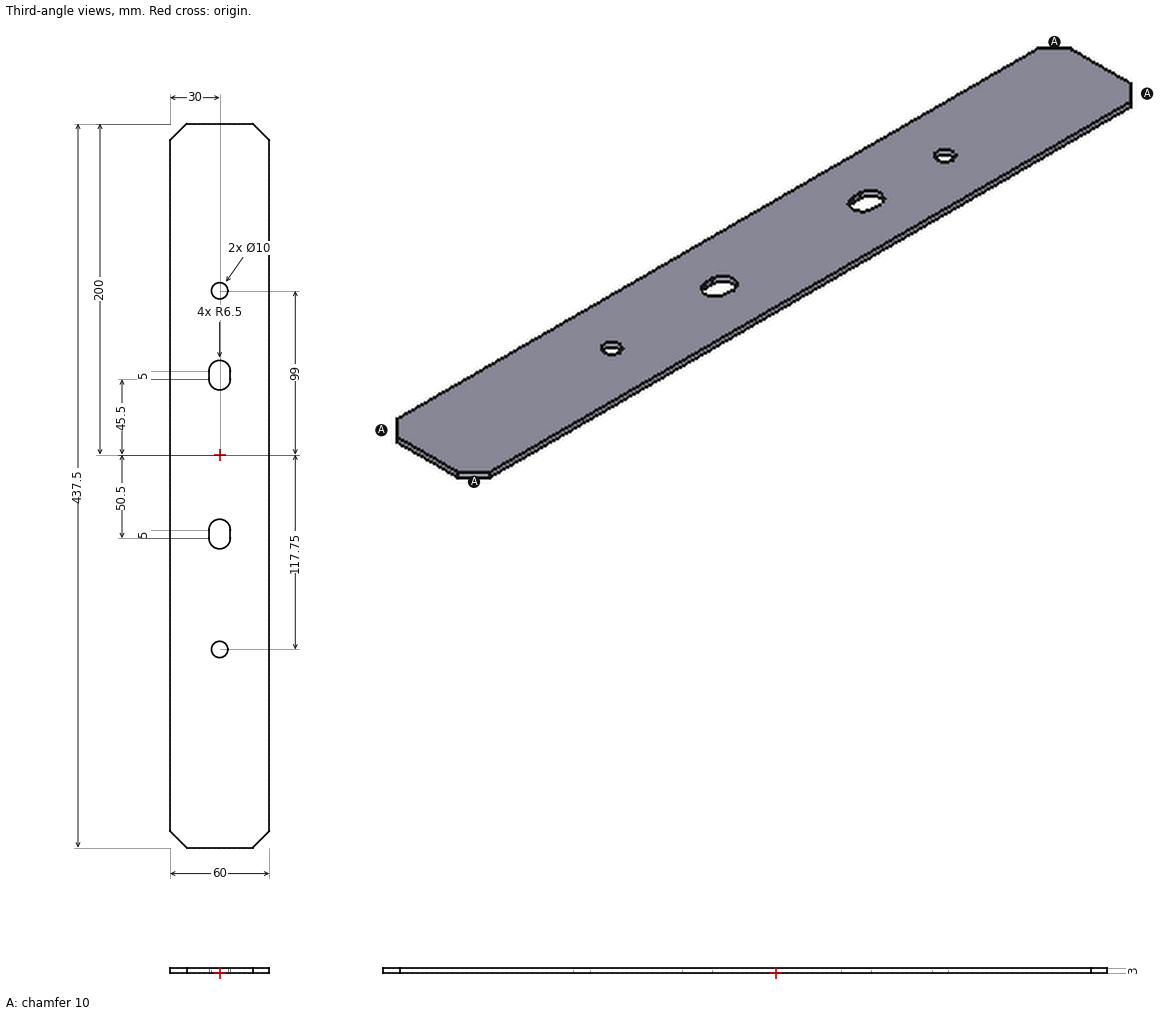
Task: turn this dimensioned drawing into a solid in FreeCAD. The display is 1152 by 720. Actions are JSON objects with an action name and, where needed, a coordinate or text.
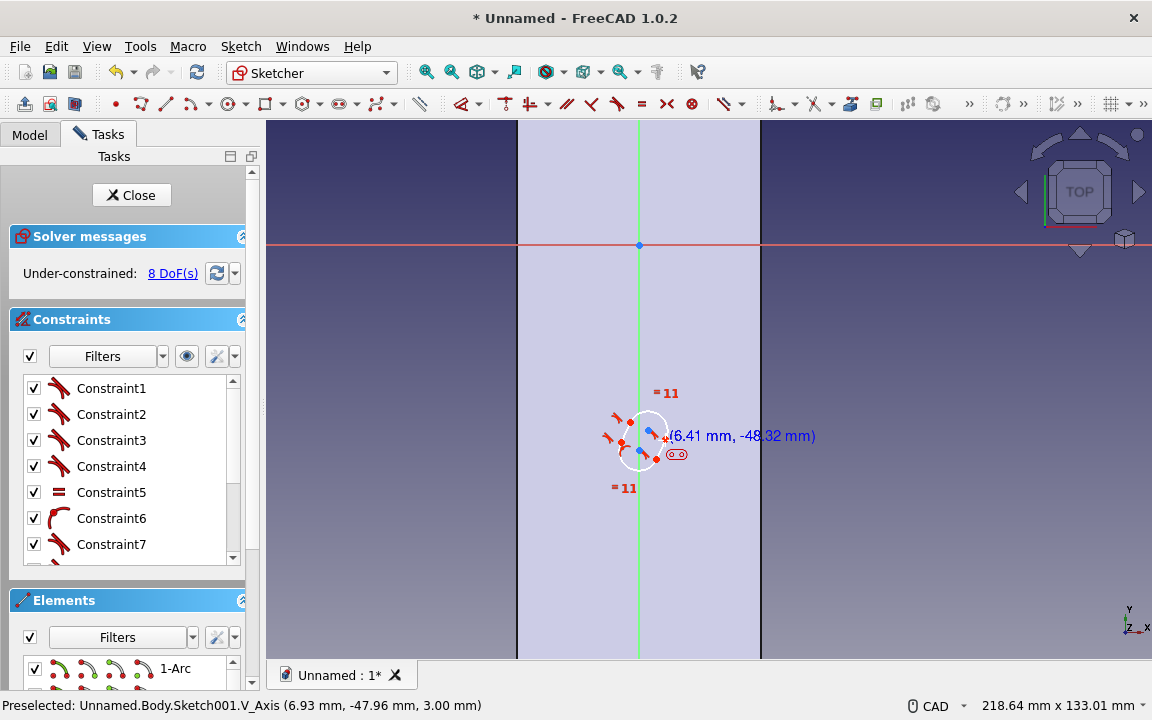
{"action": "key", "text": "g c"}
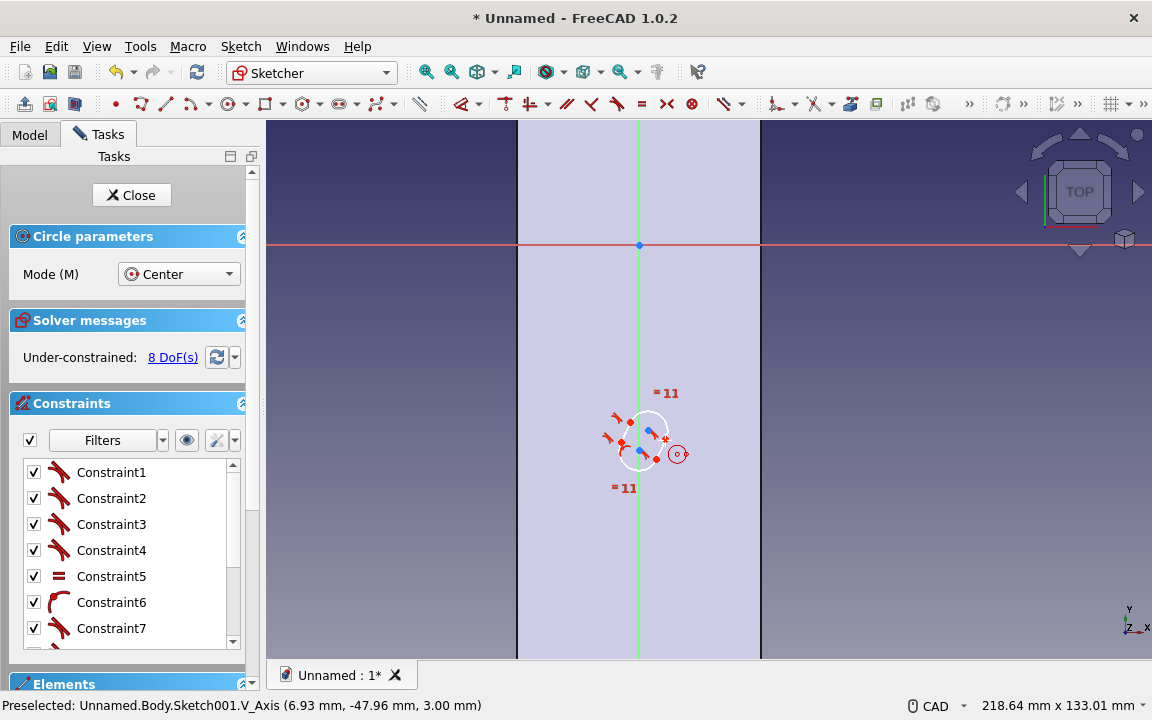
{"action": "scroll", "coordinate": [641, 451], "scroll_direction": "down", "scroll_amount": 5}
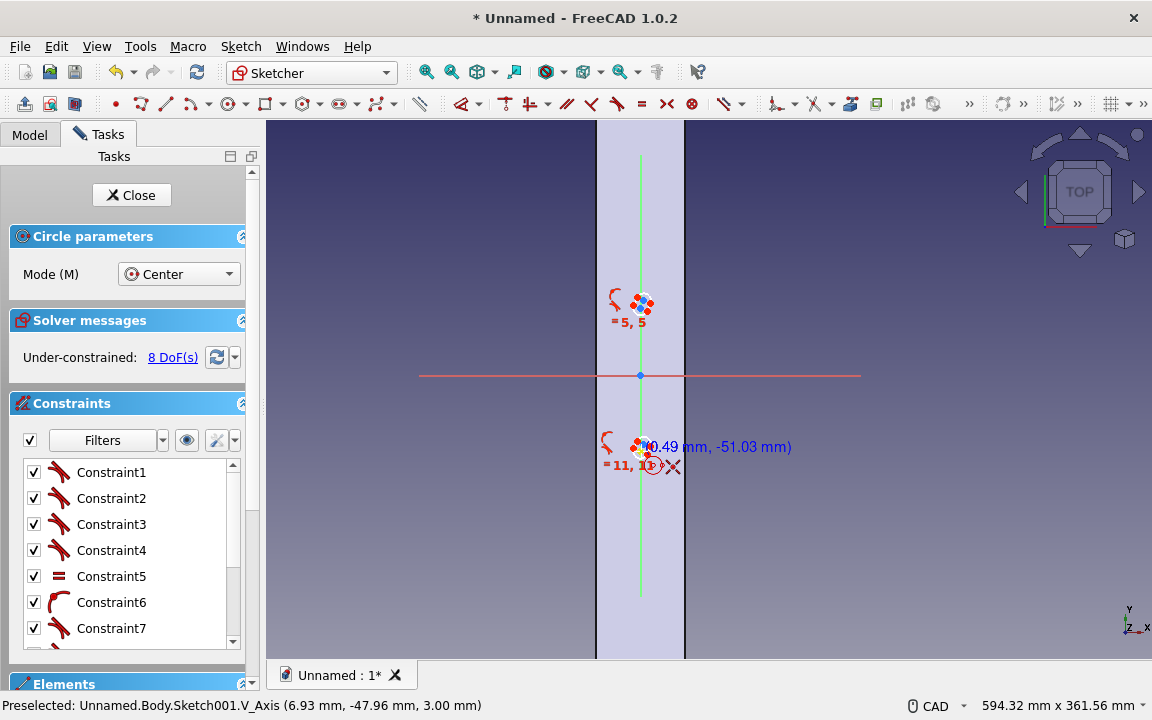
{"action": "scroll", "coordinate": [641, 228], "scroll_direction": "up", "scroll_amount": 6}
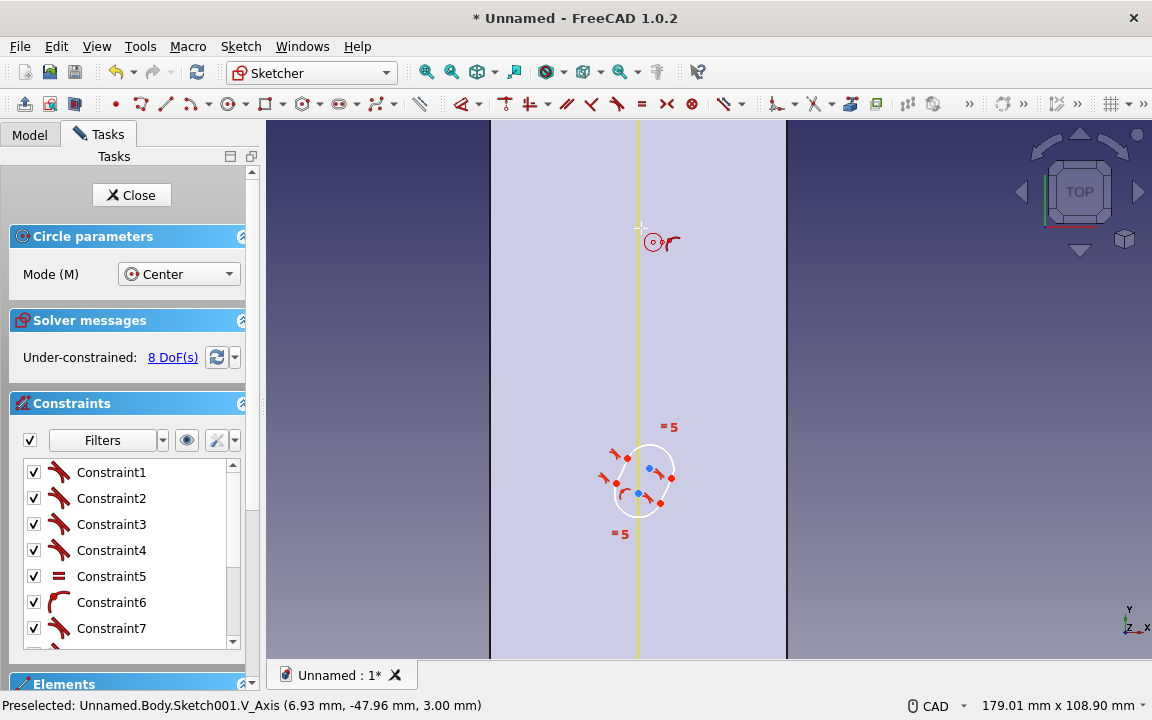
{"action": "scroll", "coordinate": [641, 228], "scroll_direction": "down", "scroll_amount": 6}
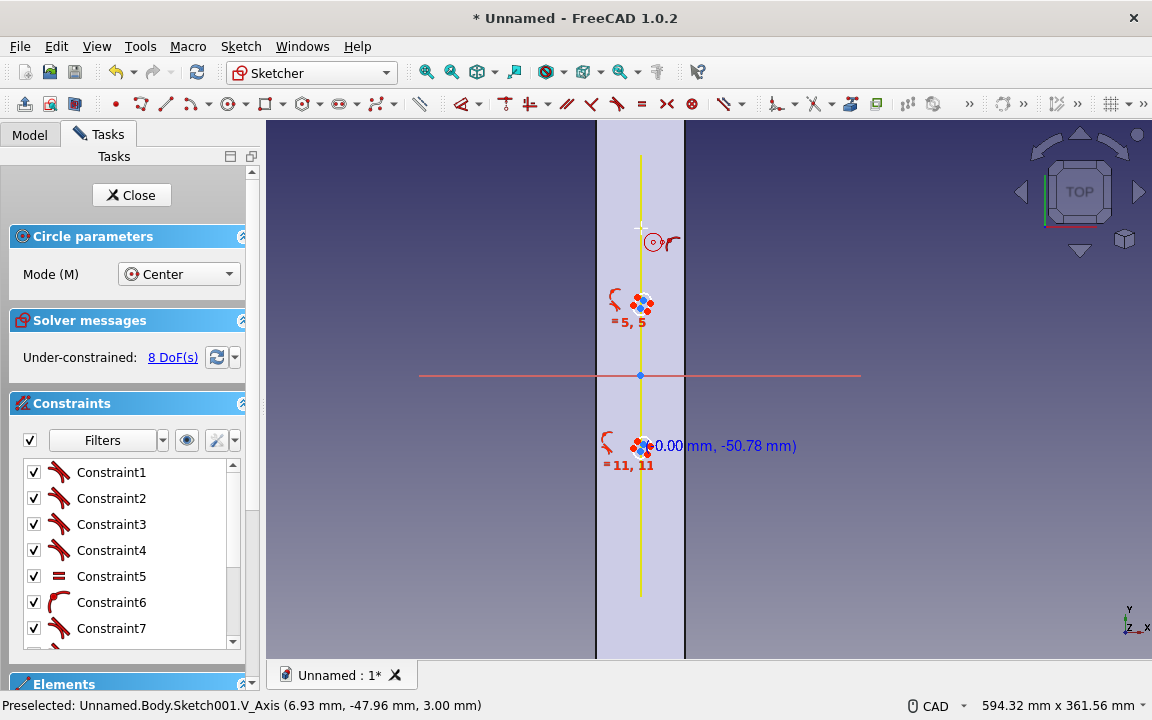
{"action": "left_click", "coordinate": [641, 228]}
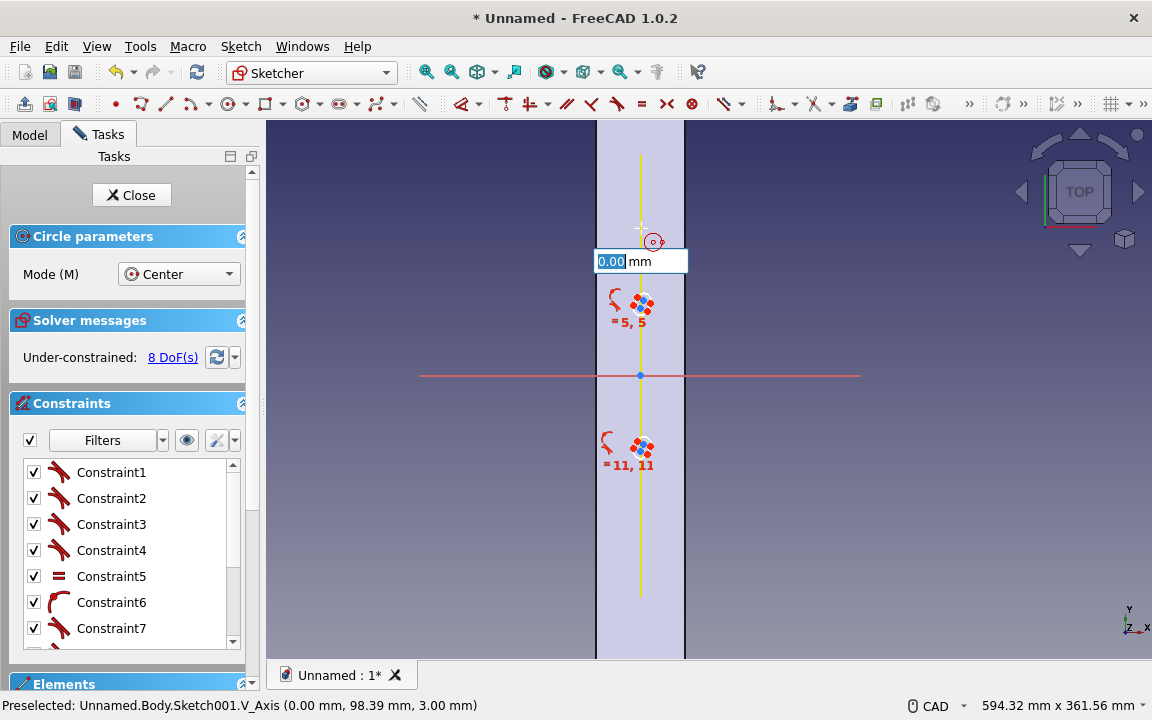
{"action": "scroll", "coordinate": [648, 226], "scroll_direction": "up", "scroll_amount": 5}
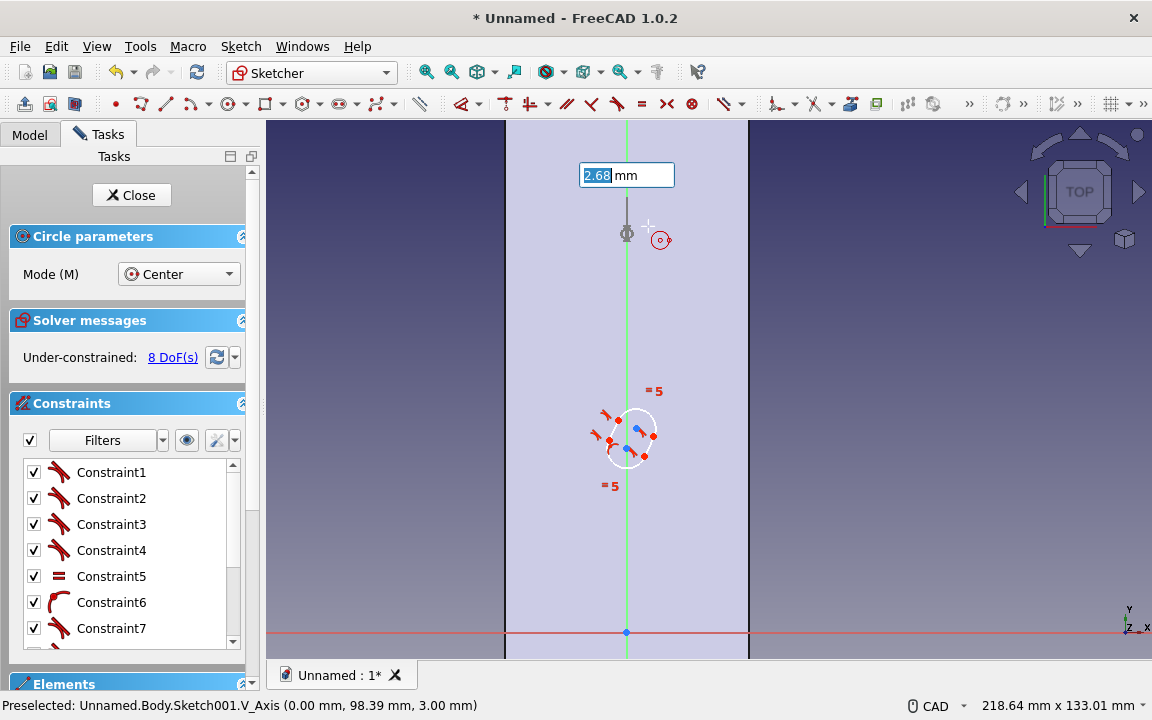
{"action": "left_click", "coordinate": [646, 224]}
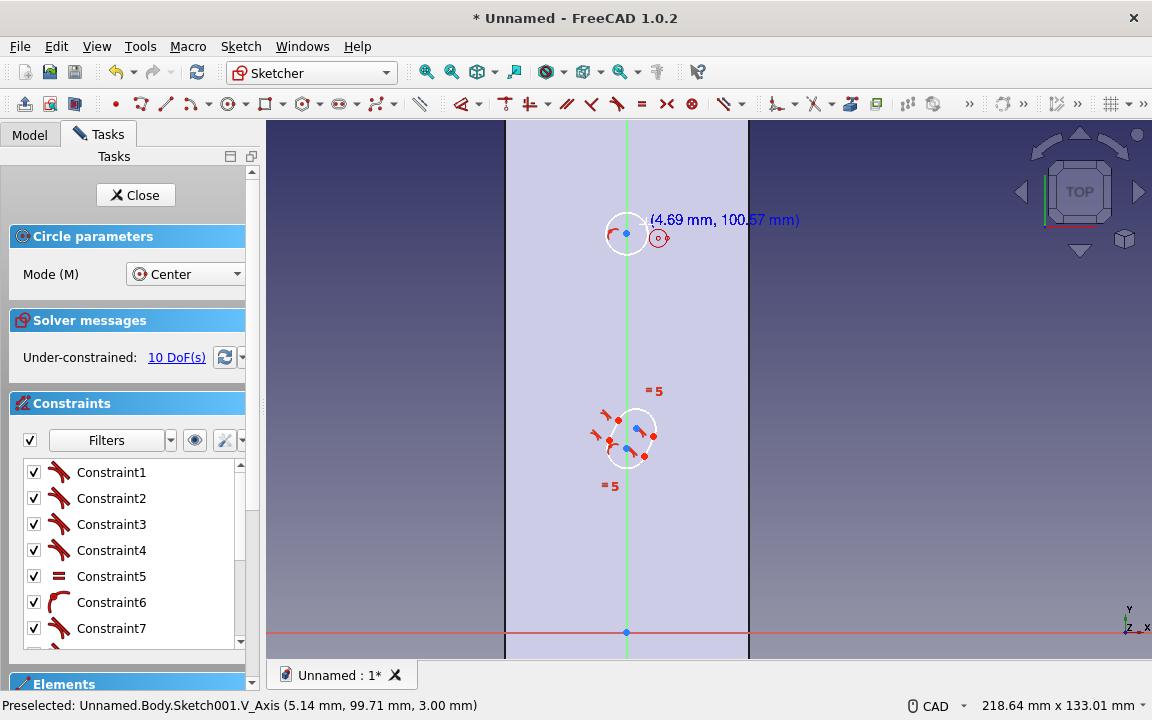
{"action": "scroll", "coordinate": [648, 226], "scroll_direction": "down", "scroll_amount": 5}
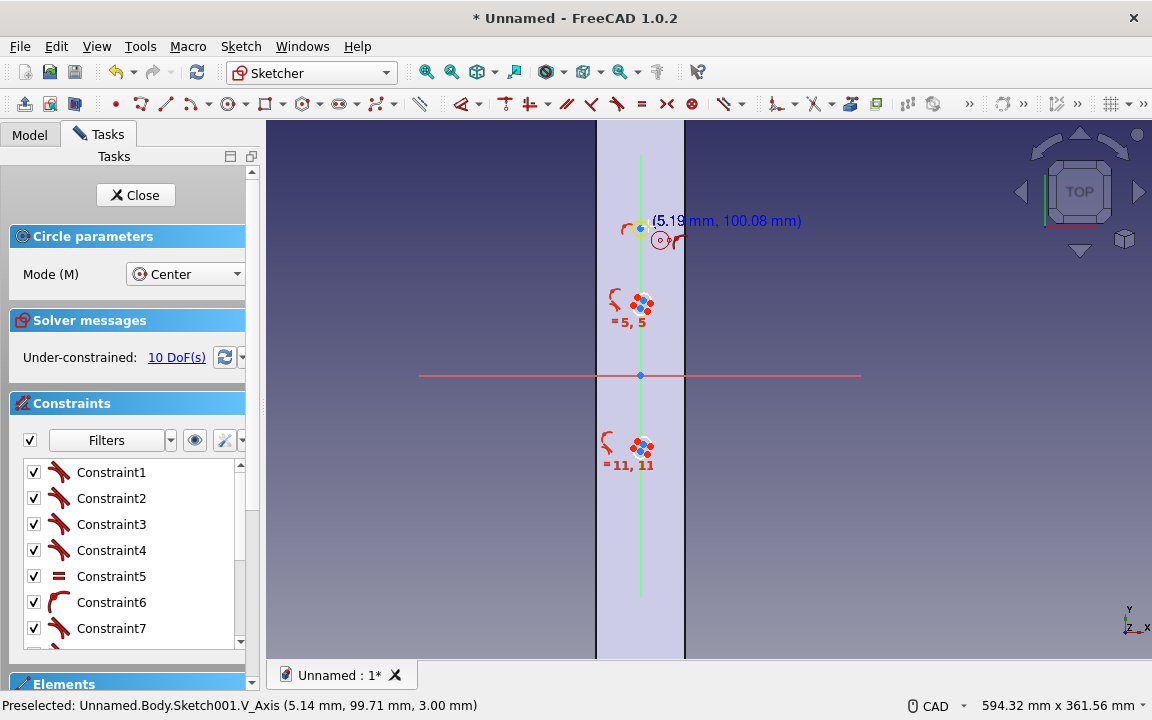
{"action": "scroll", "coordinate": [641, 551], "scroll_direction": "up", "scroll_amount": 6}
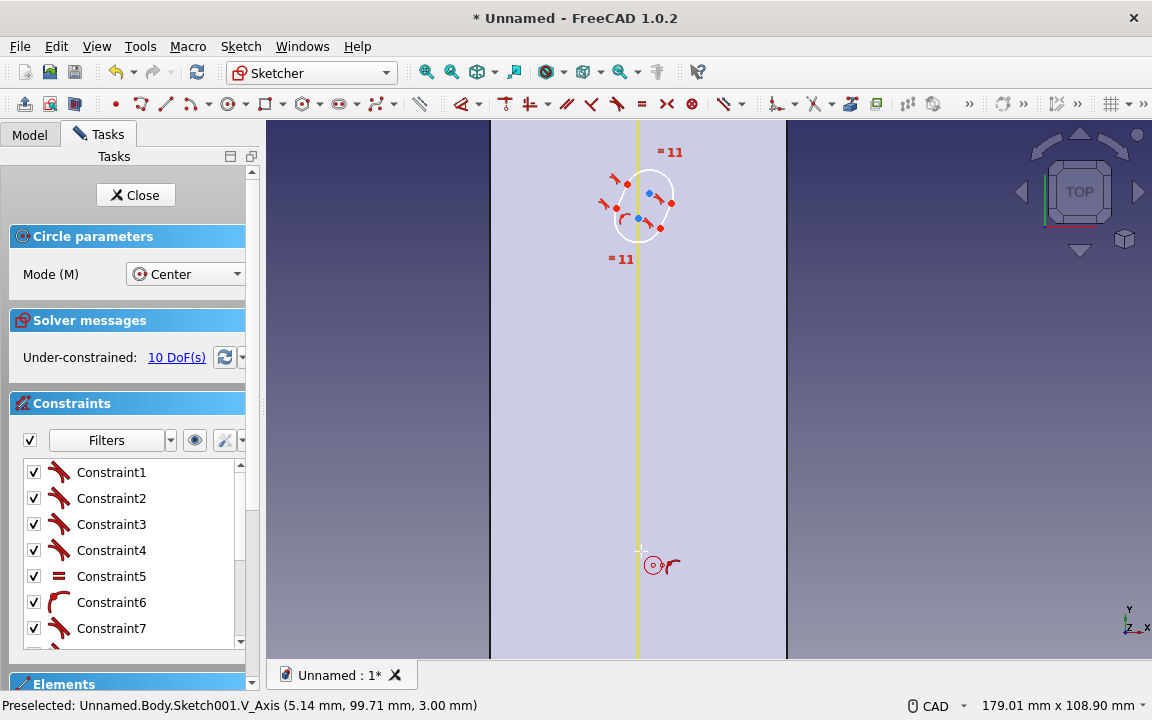
{"action": "scroll", "coordinate": [641, 552], "scroll_direction": "down", "scroll_amount": 6}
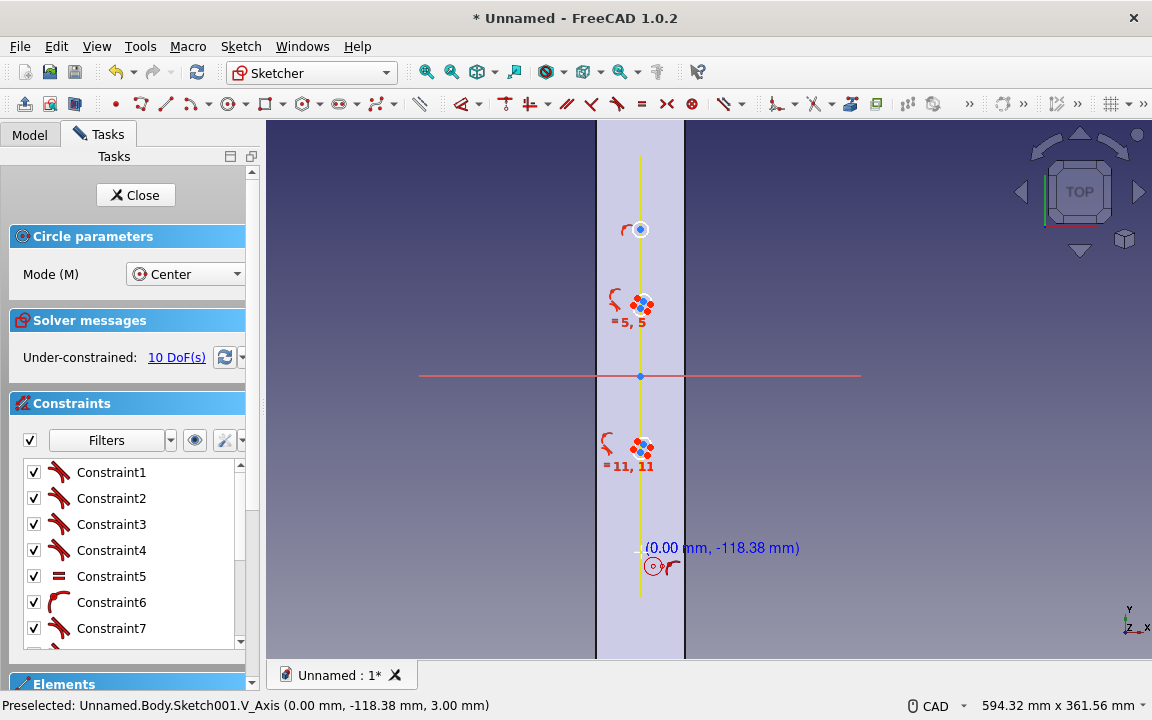
{"action": "left_click", "coordinate": [641, 552]}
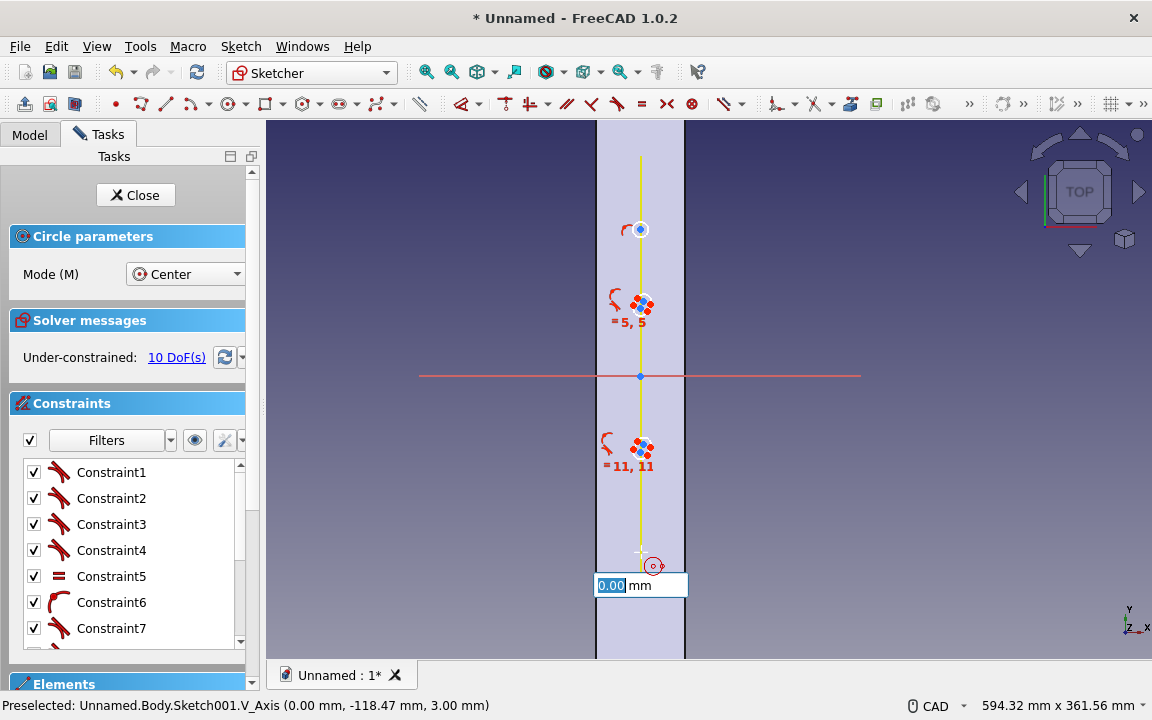
{"action": "scroll", "coordinate": [648, 549], "scroll_direction": "up", "scroll_amount": 5}